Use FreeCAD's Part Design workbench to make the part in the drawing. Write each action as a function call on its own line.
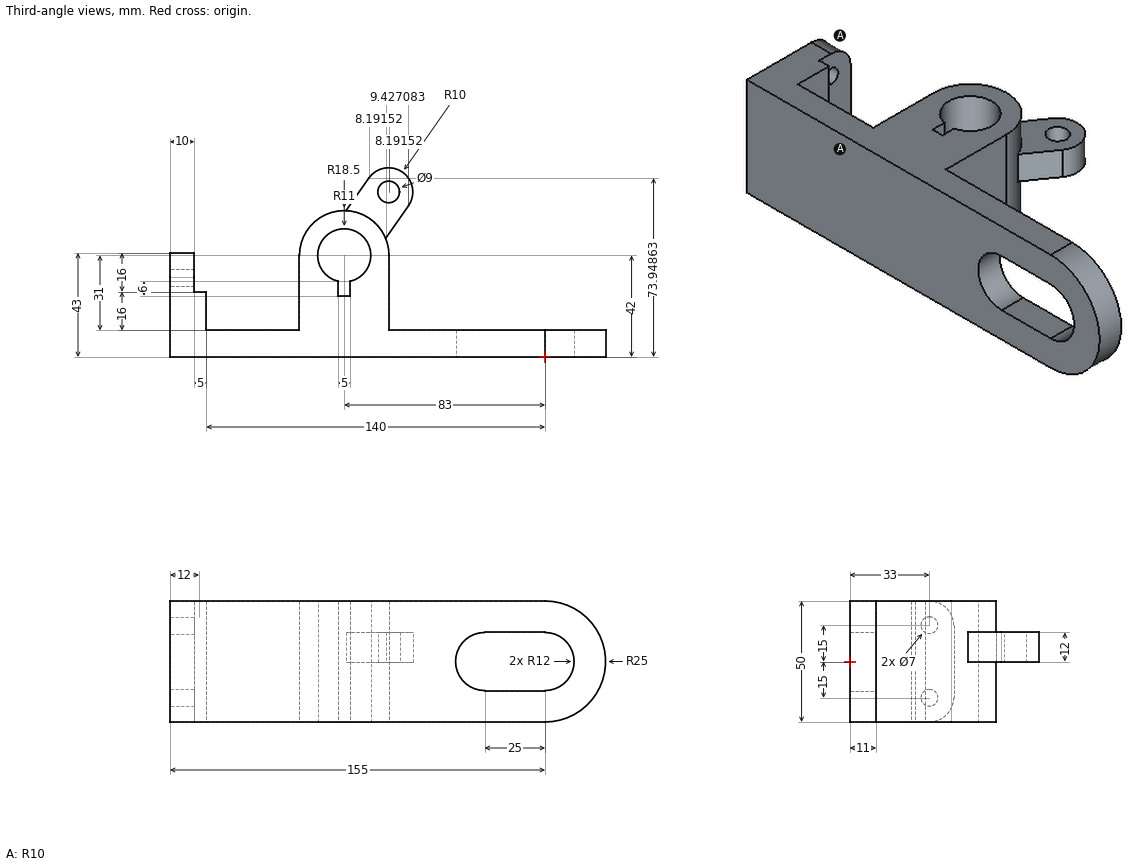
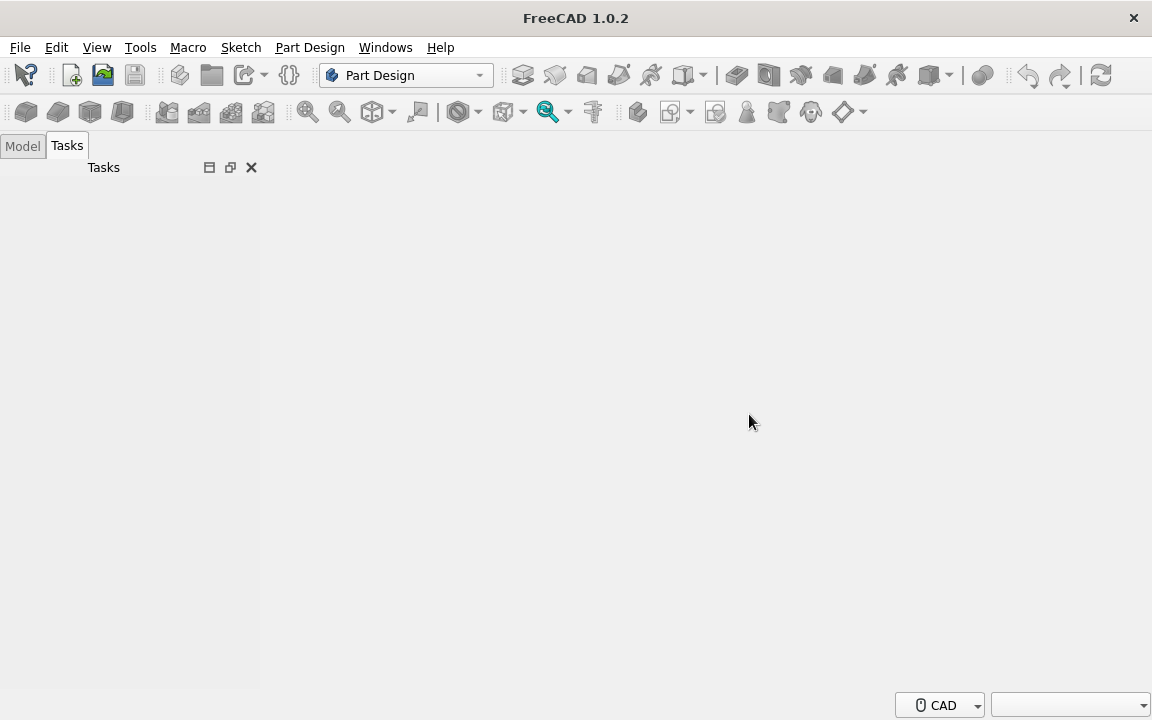
click(72, 76)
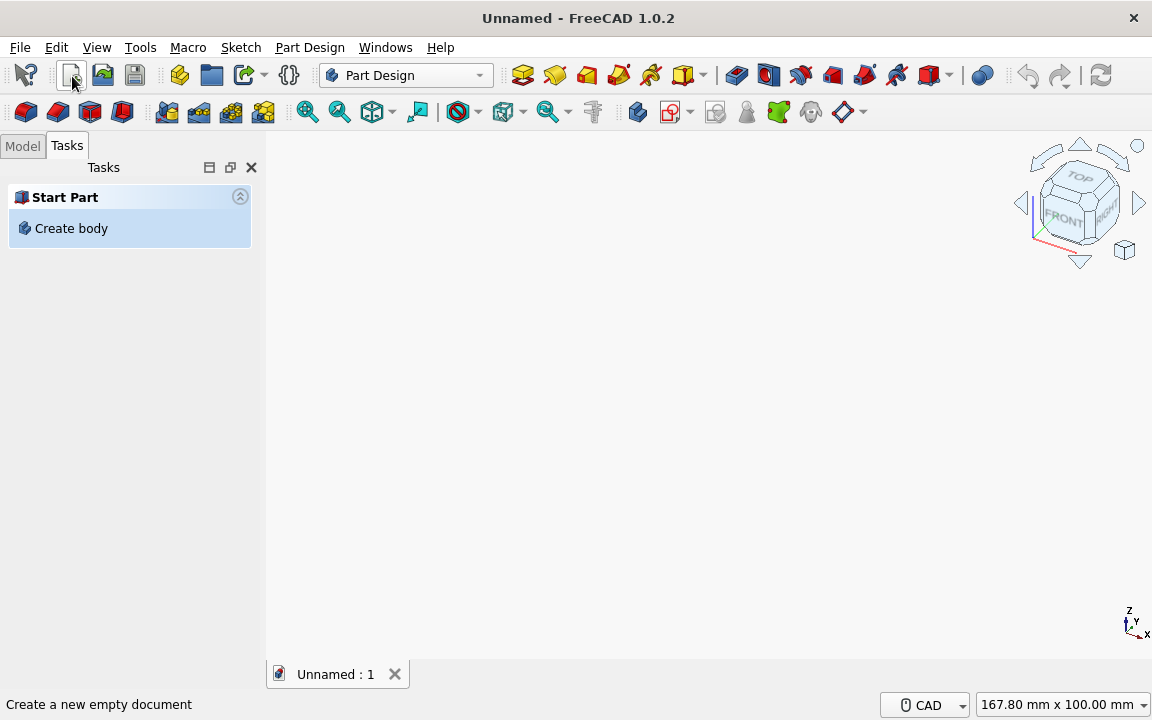
click(670, 112)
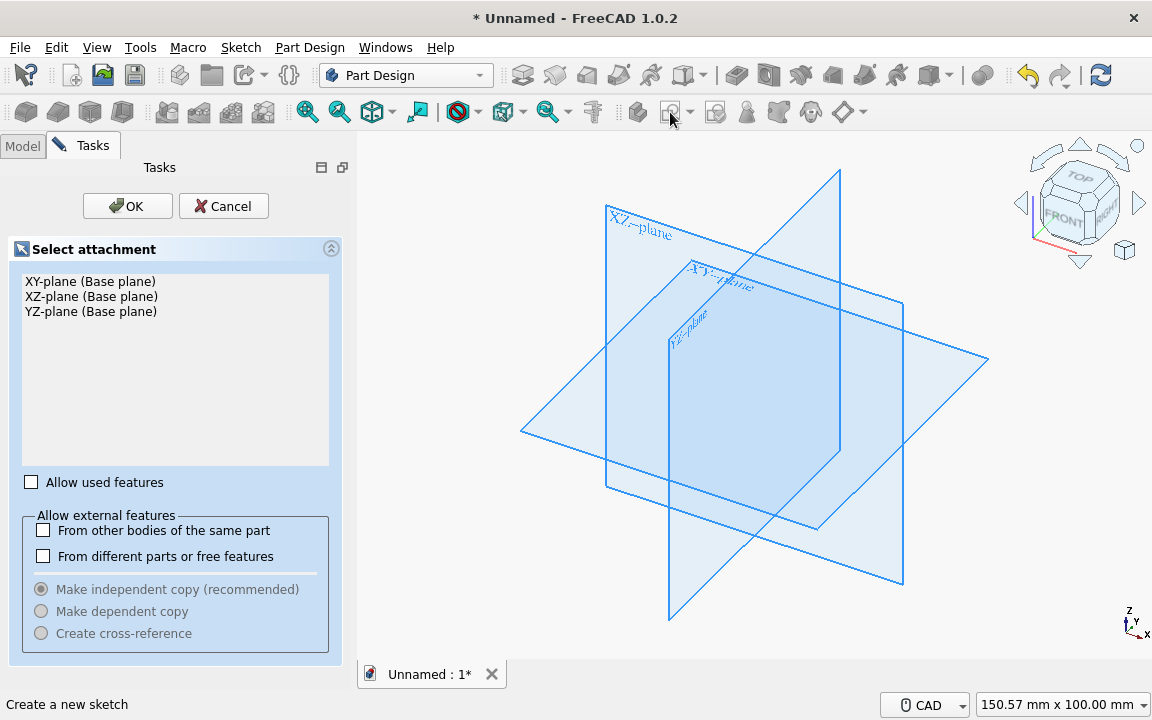
click(82, 296)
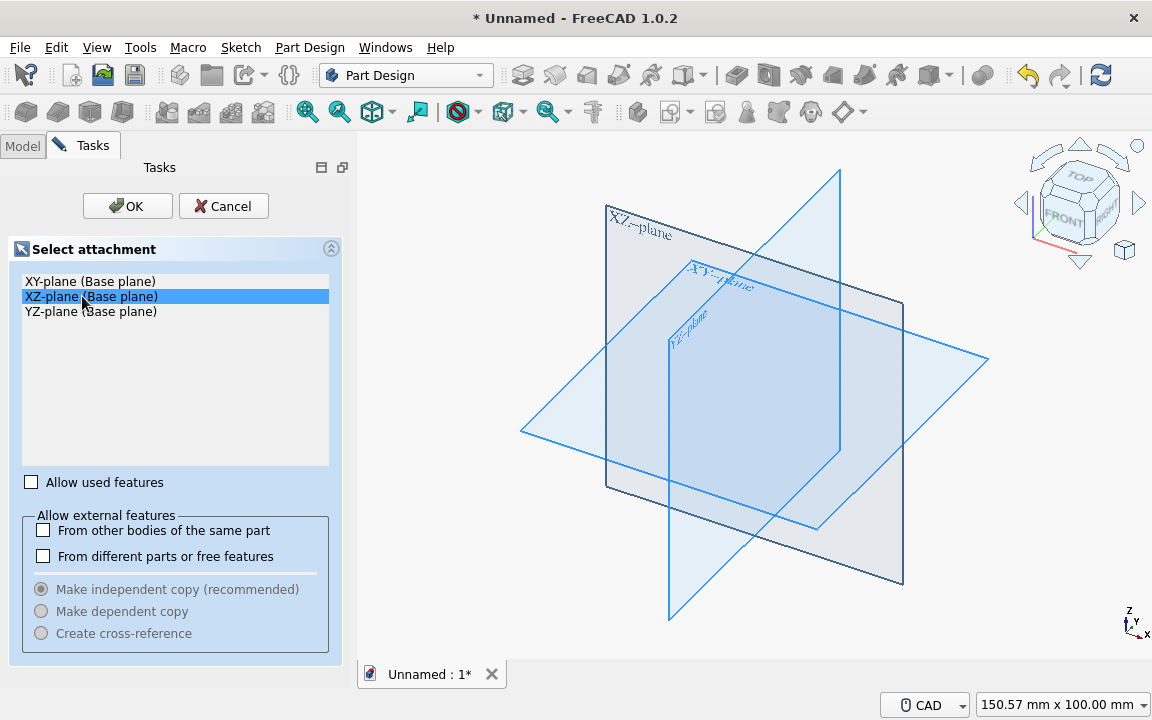
click(128, 206)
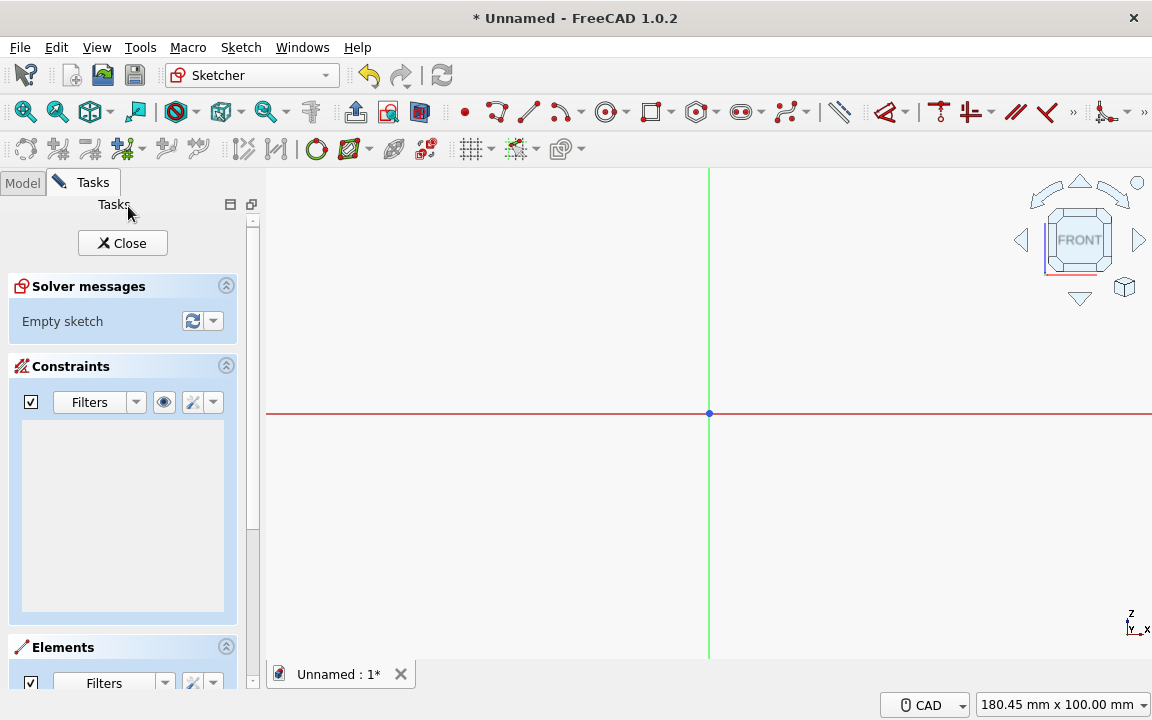
scroll(945, 414, down, 3)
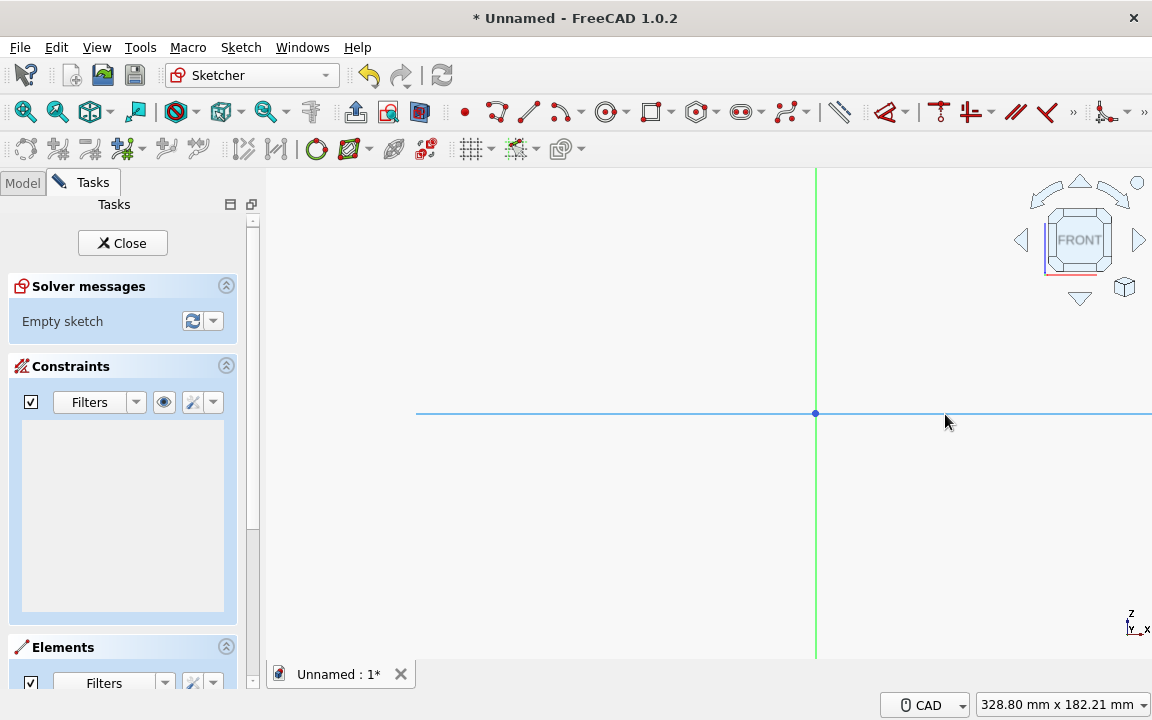
click(498, 112)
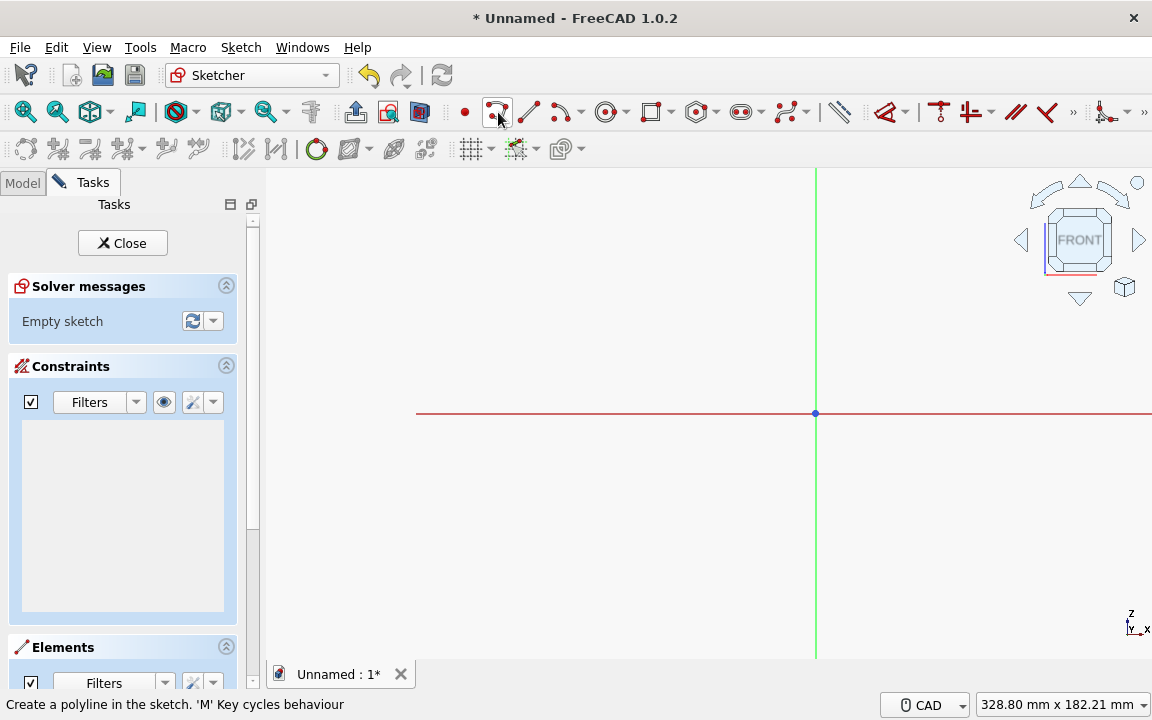
click(816, 481)
click(398, 481)
click(398, 347)
click(816, 347)
right_click(816, 347)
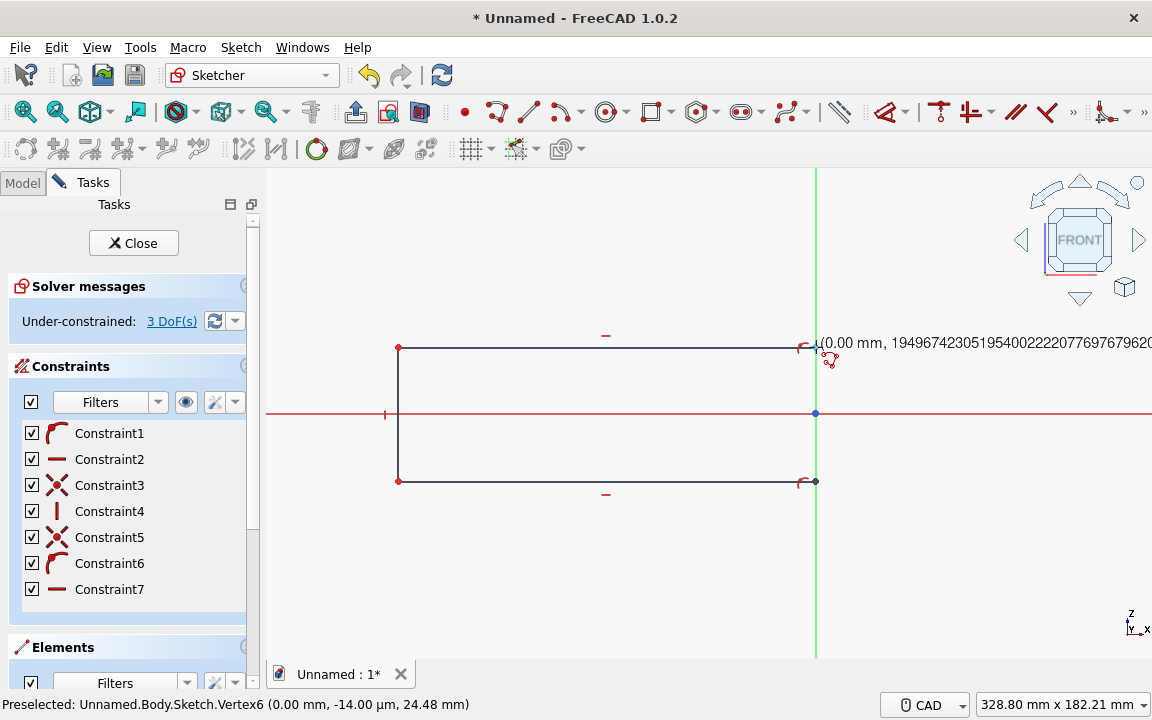
key(g)
key(3)
key(a)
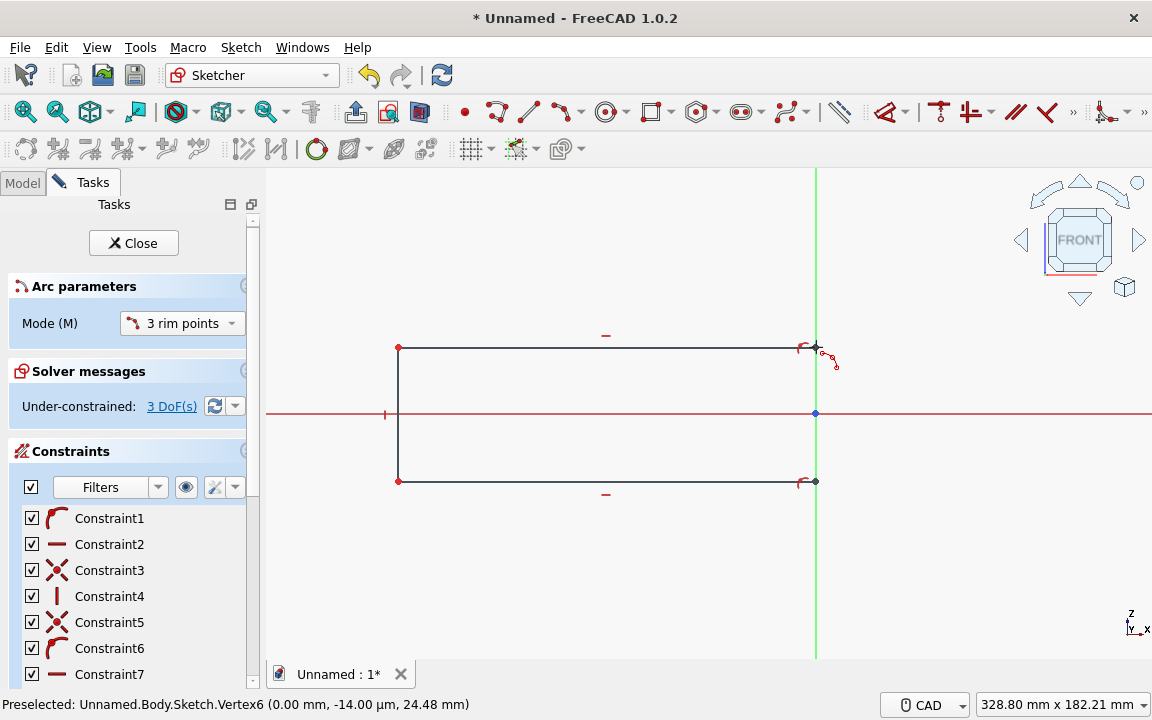
click(816, 348)
click(816, 482)
click(880, 435)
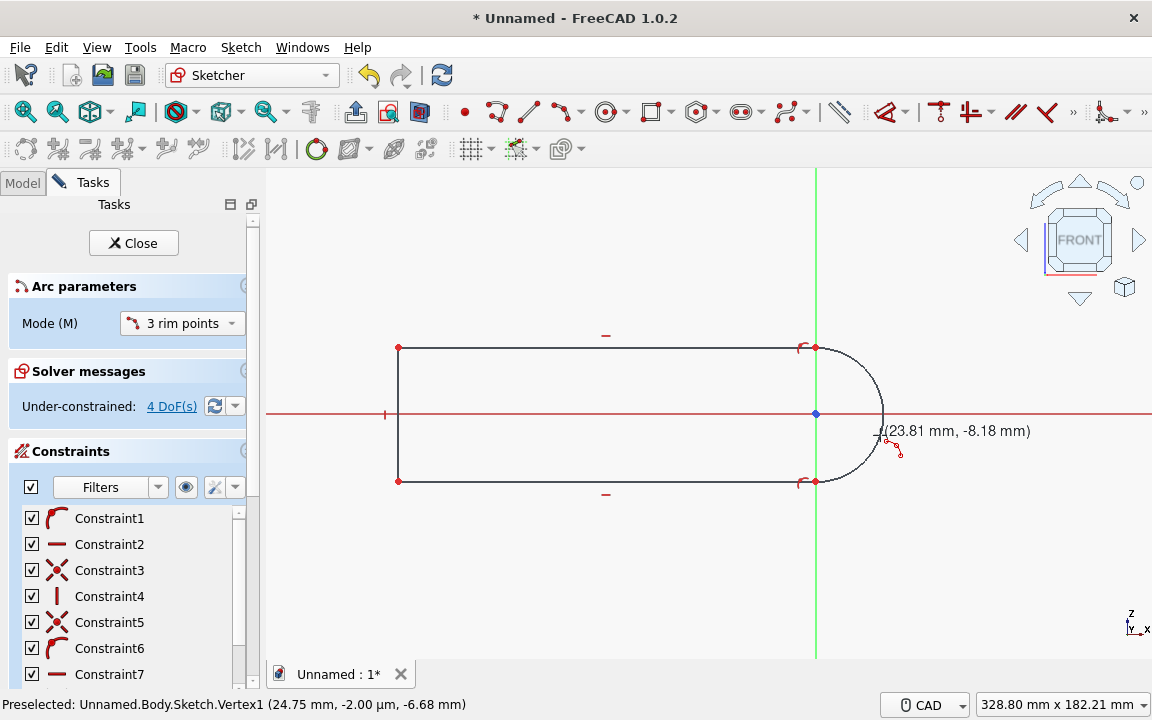
click(742, 112)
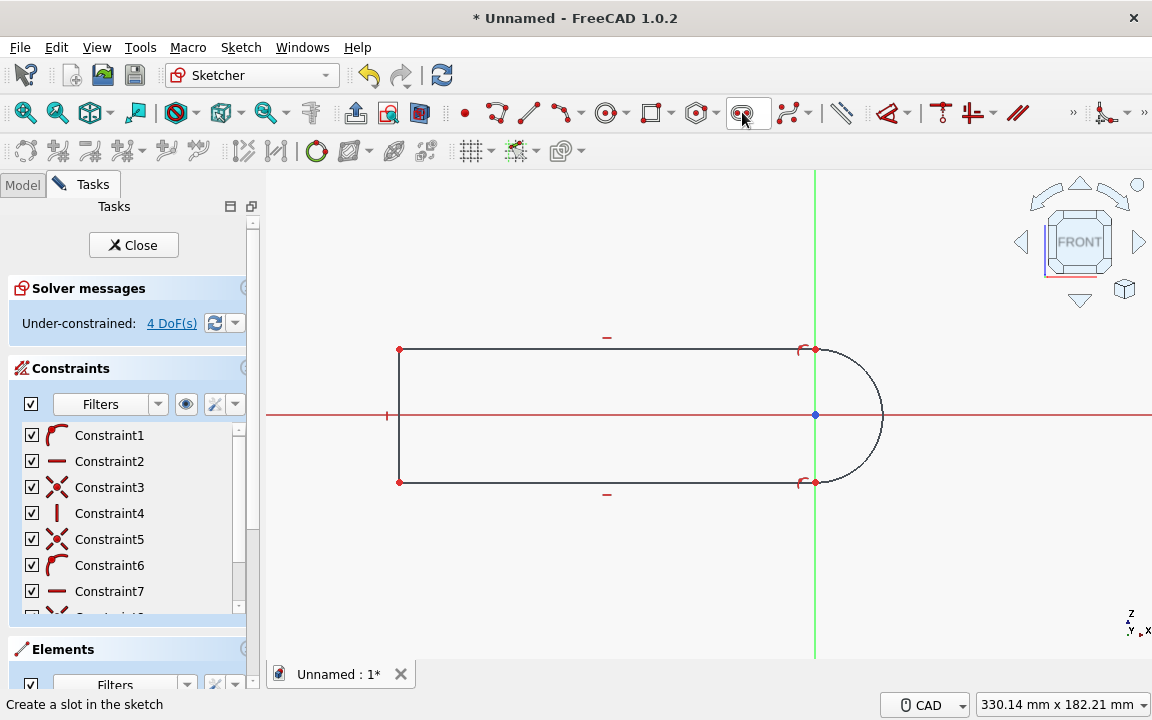
click(815, 415)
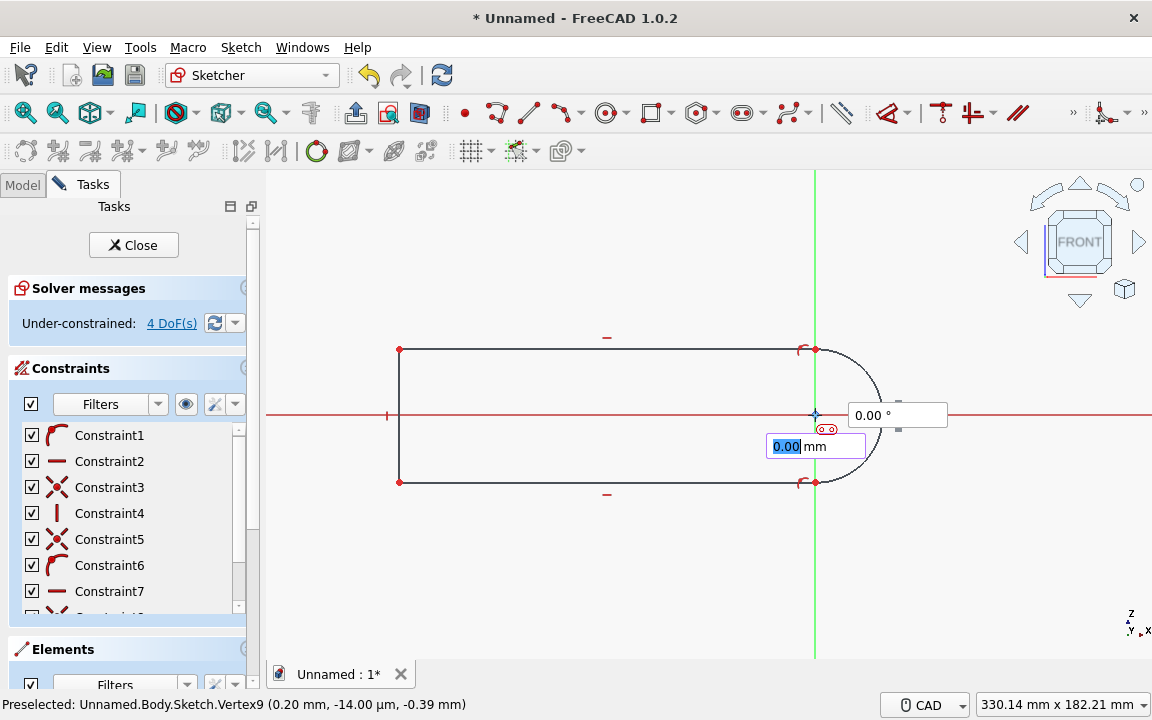
click(748, 406)